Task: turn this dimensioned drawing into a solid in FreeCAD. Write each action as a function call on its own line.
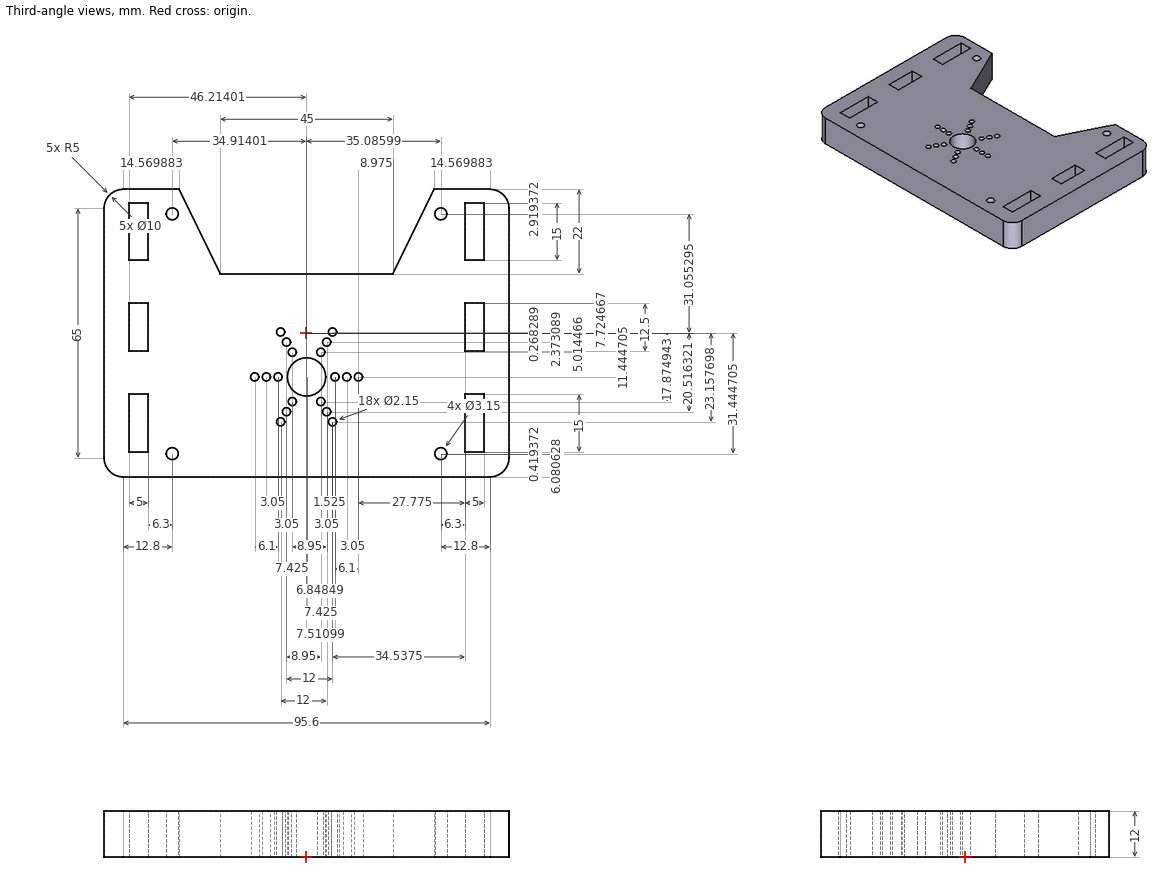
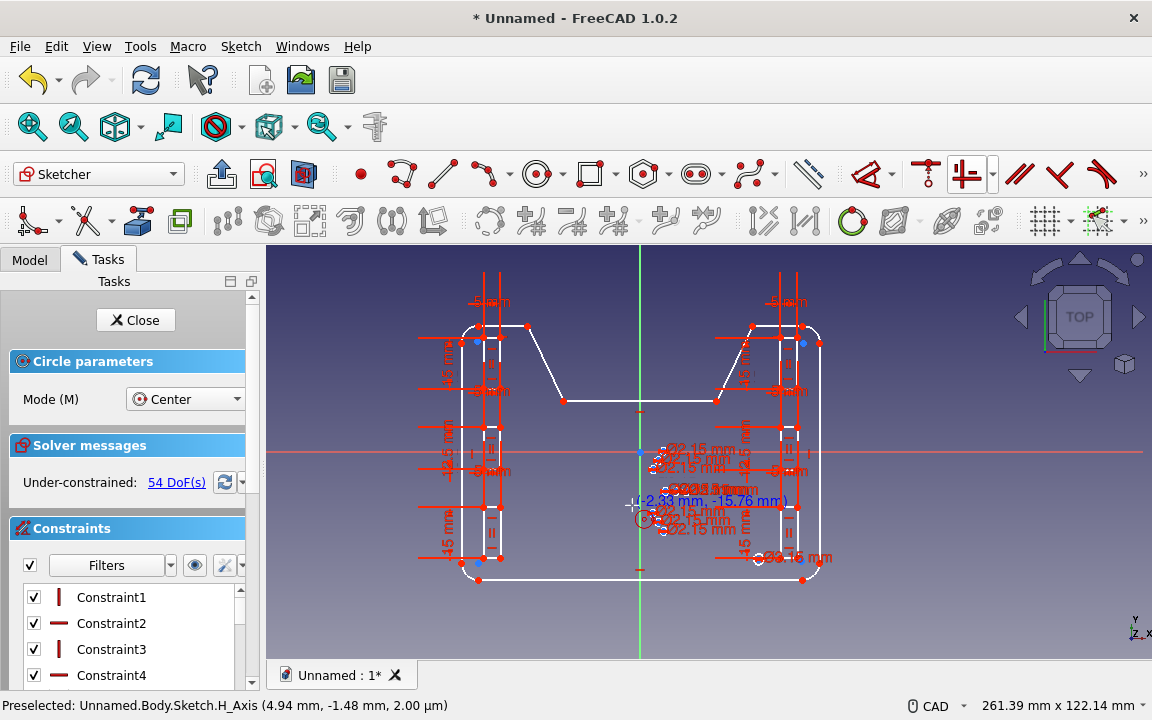
click(623, 522)
move(625, 519)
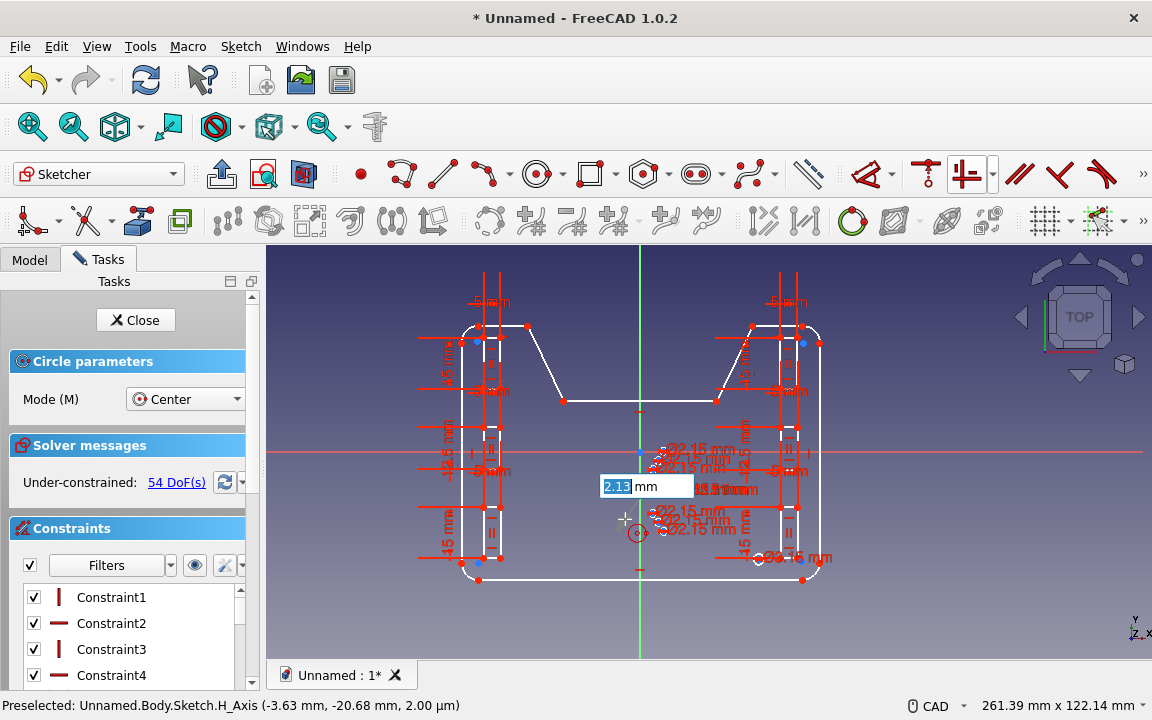
text(2.15)
key(Return)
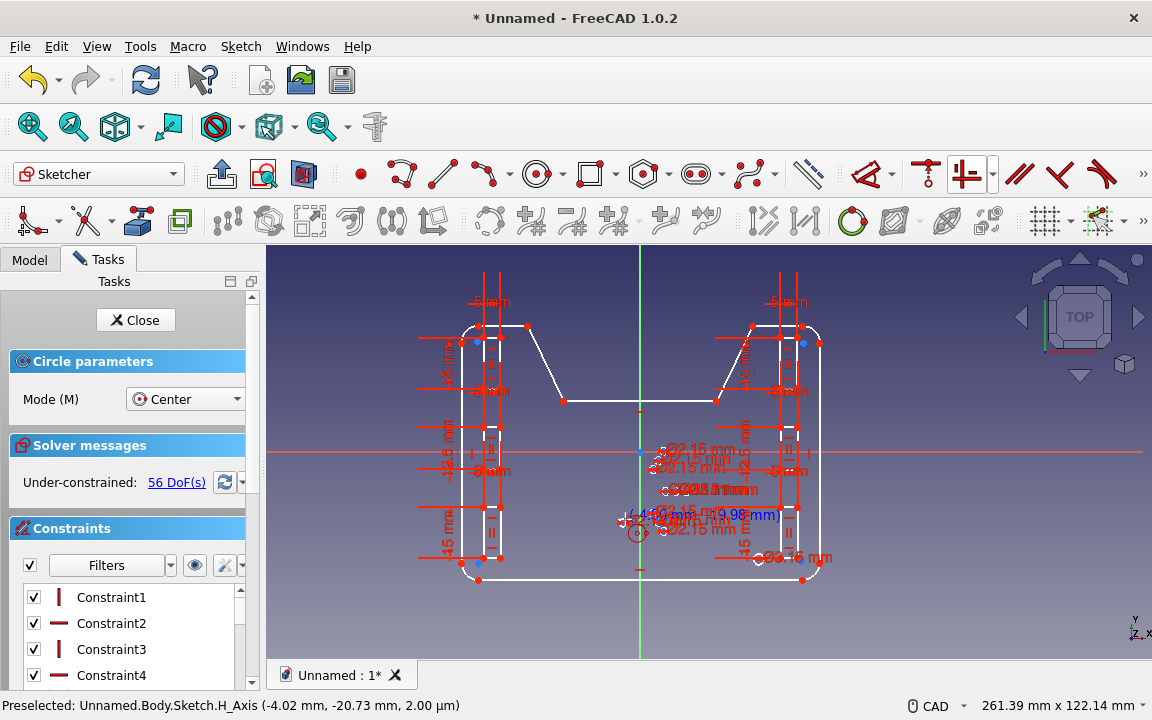
scroll(618, 531, up, 10)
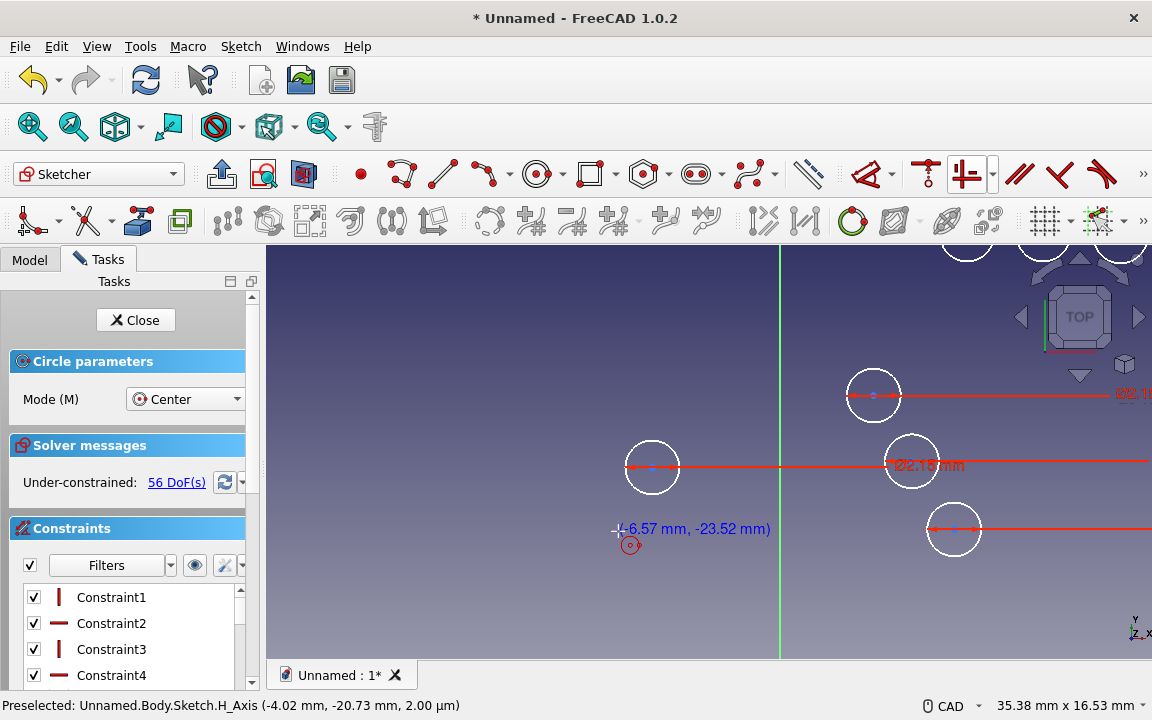
scroll(618, 531, down, 10)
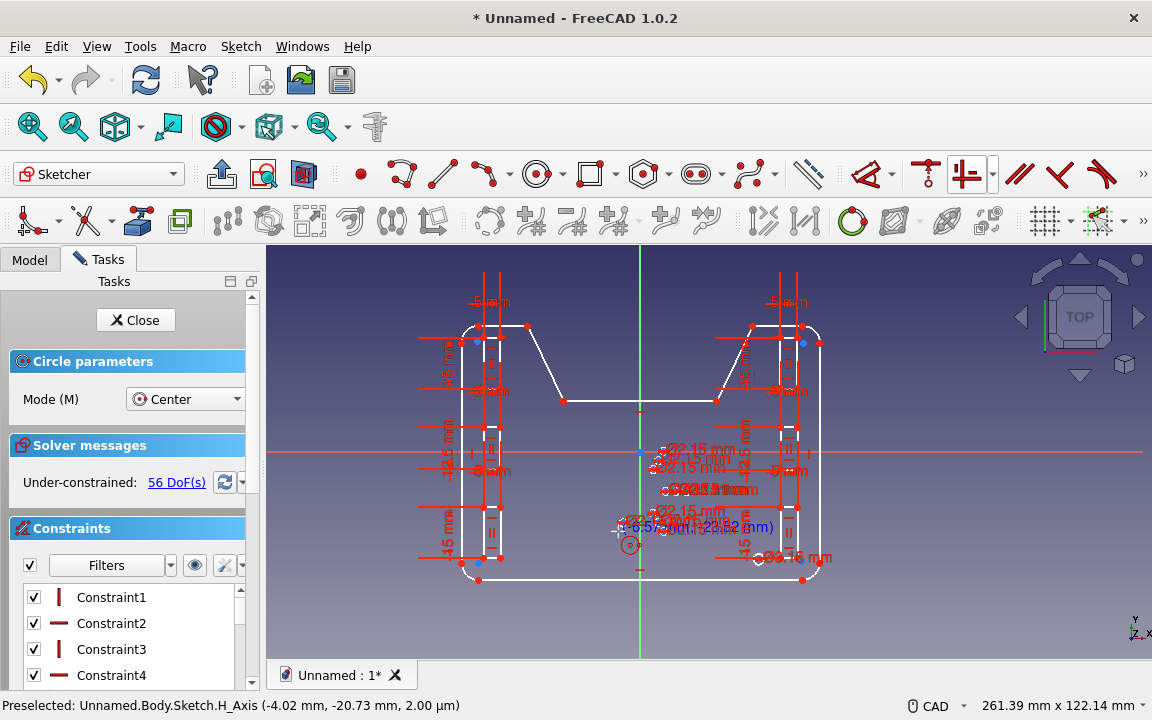
scroll(618, 531, up, 5)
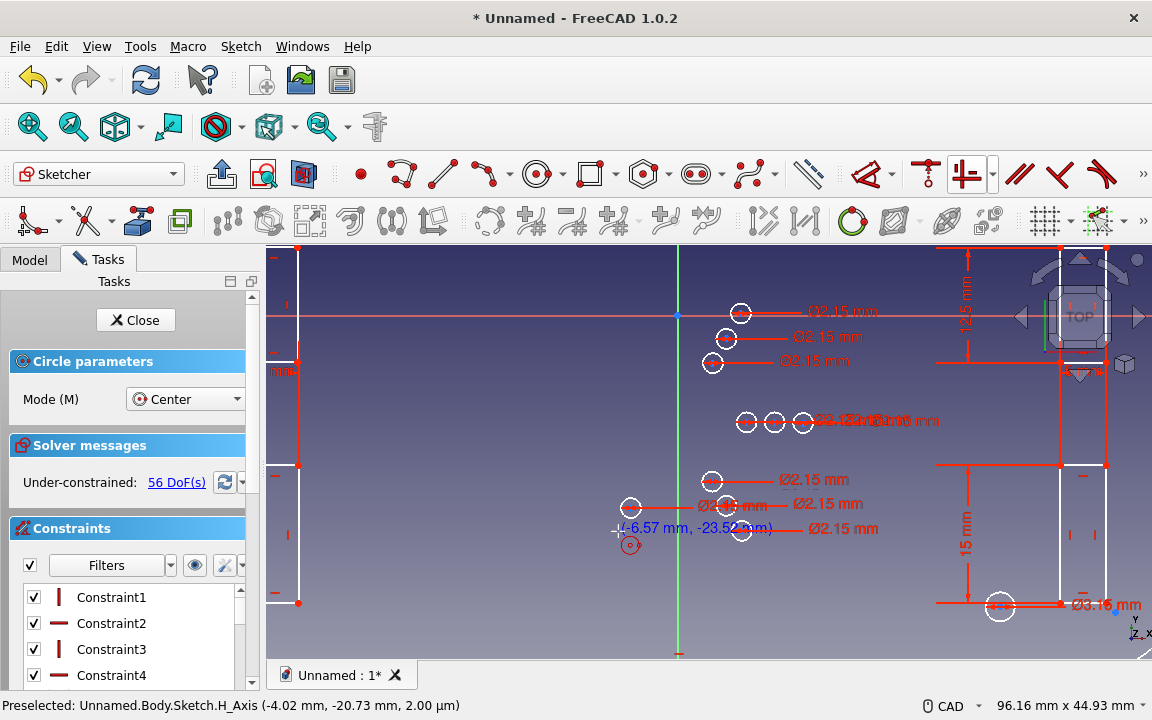
click(616, 529)
move(609, 522)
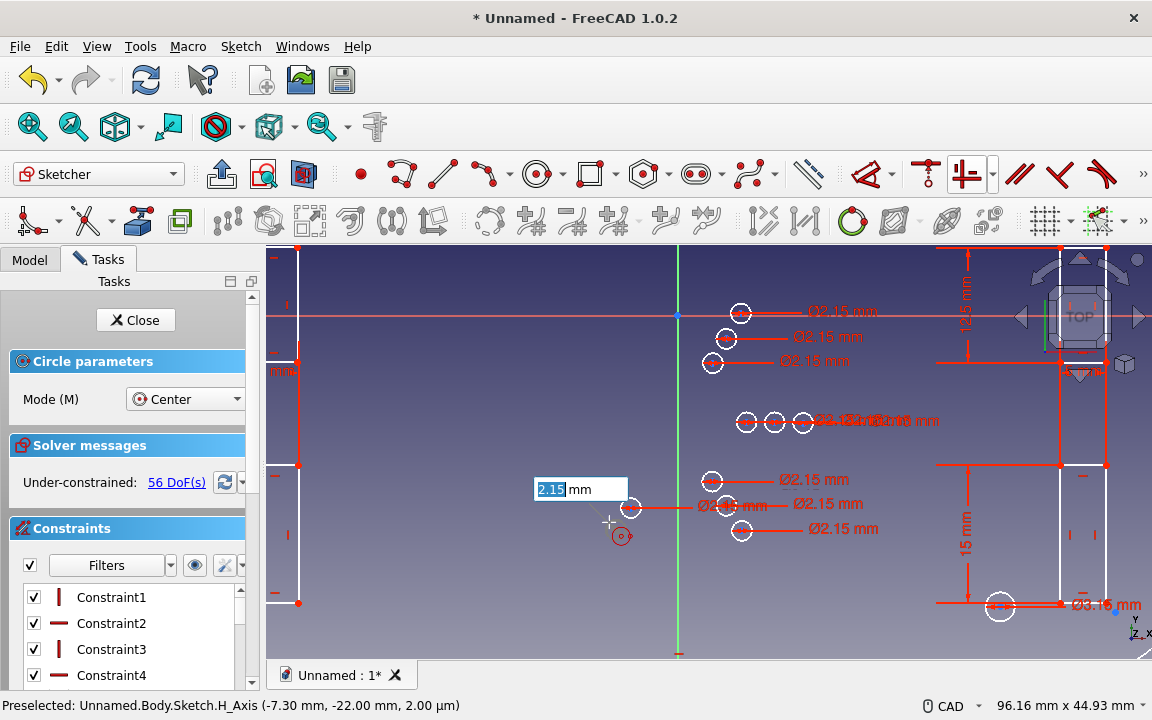
text(2.15)
key(Return)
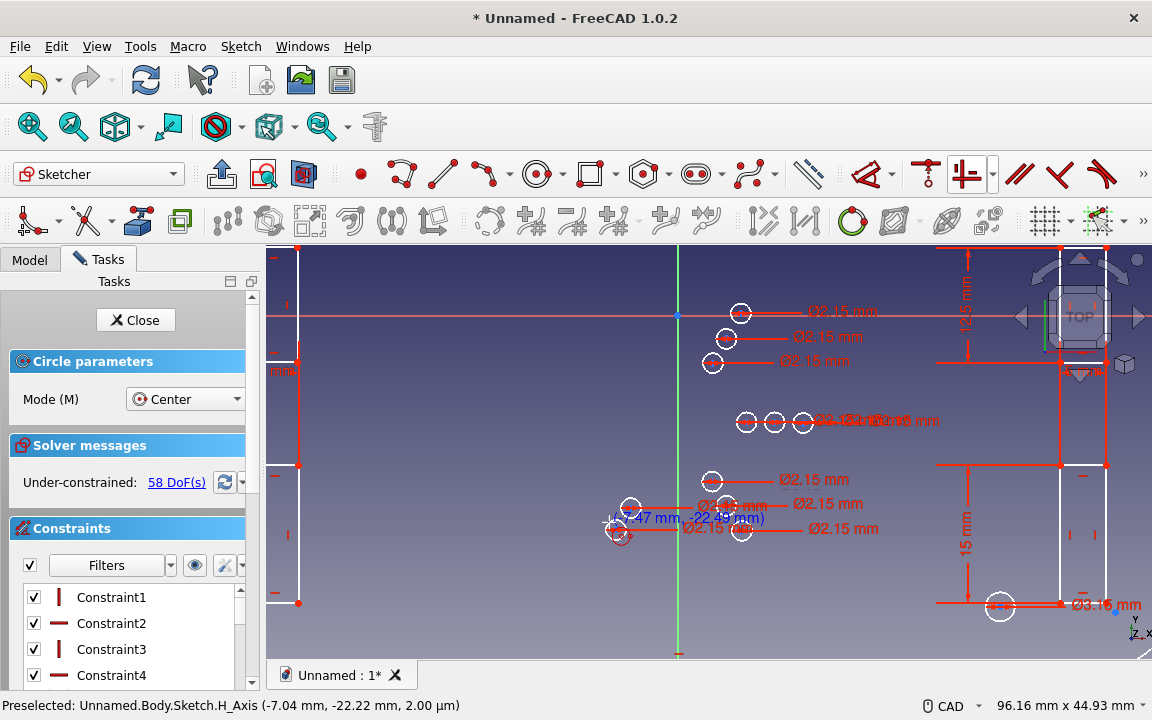
scroll(644, 481, up, 5)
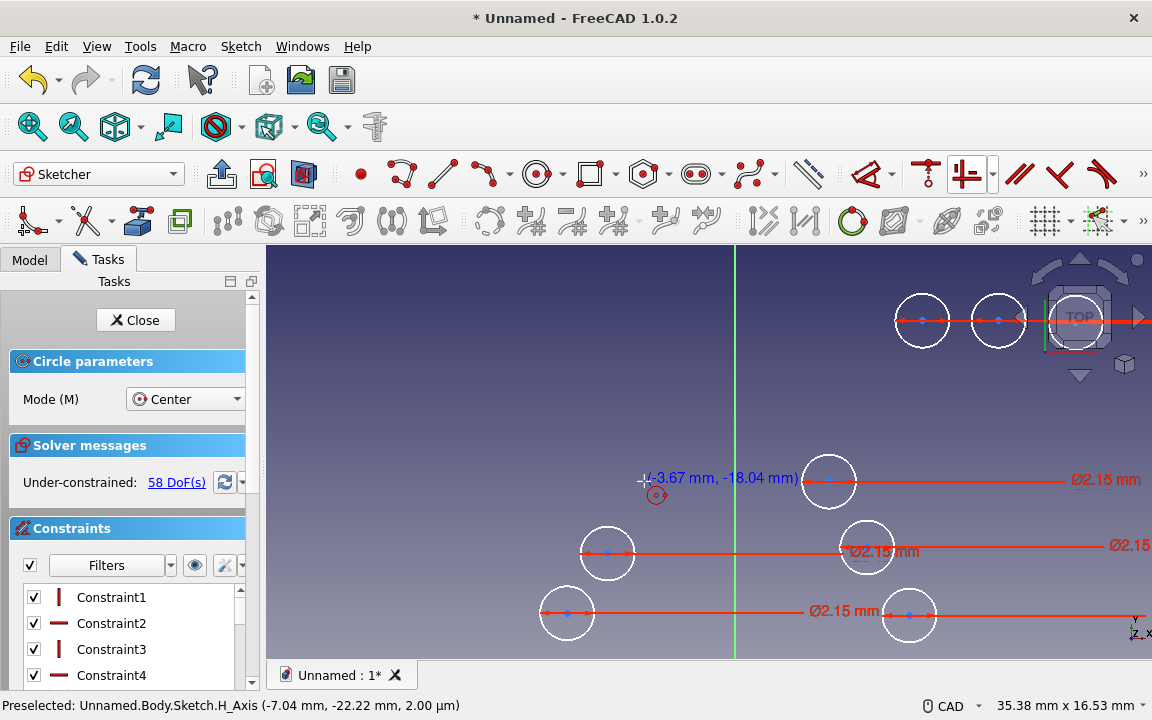
scroll(625, 518, down, 10)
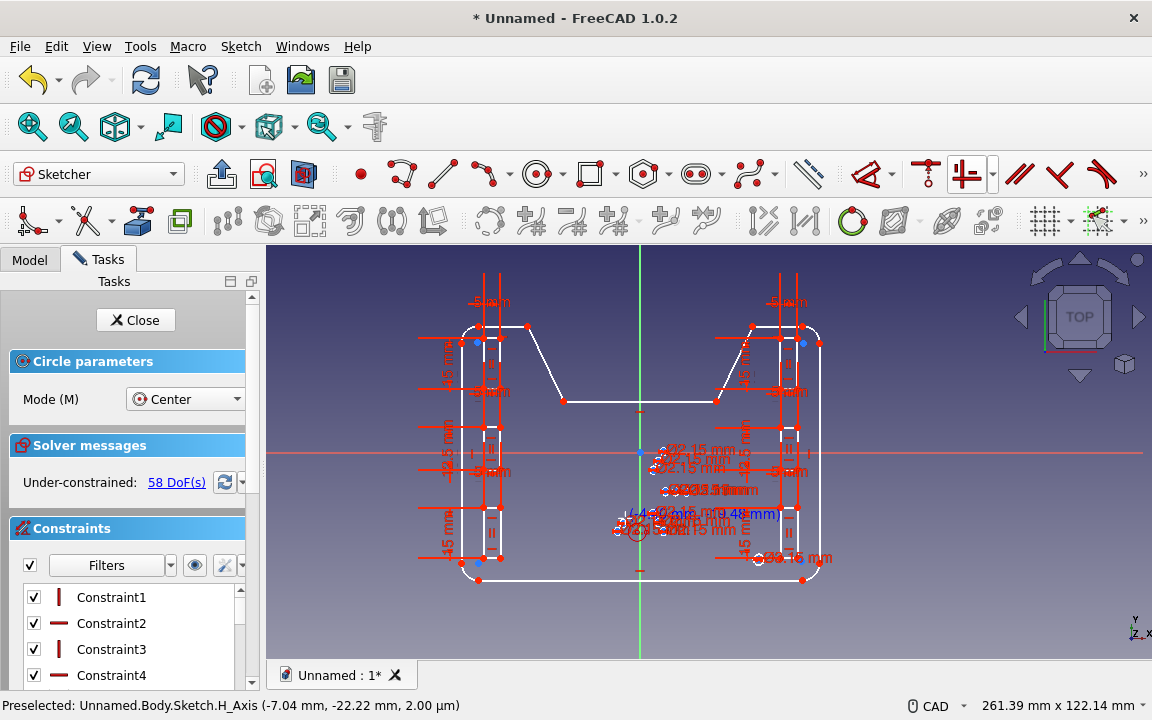
scroll(628, 513, up, 5)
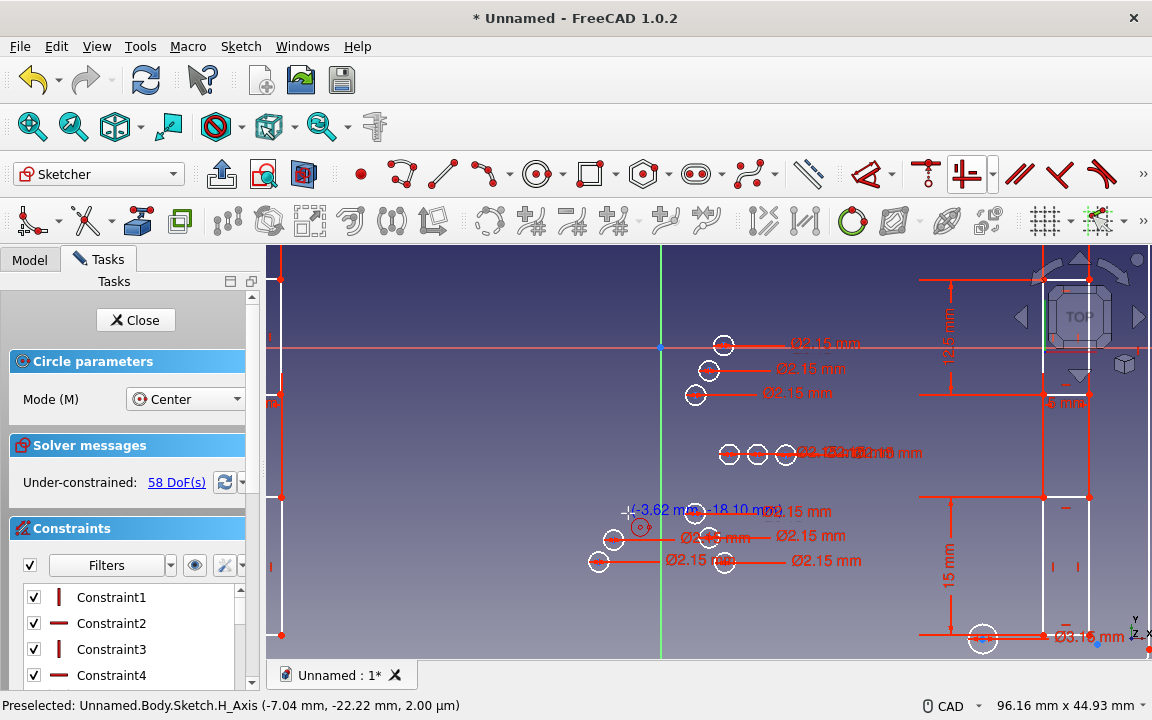
click(627, 513)
move(634, 506)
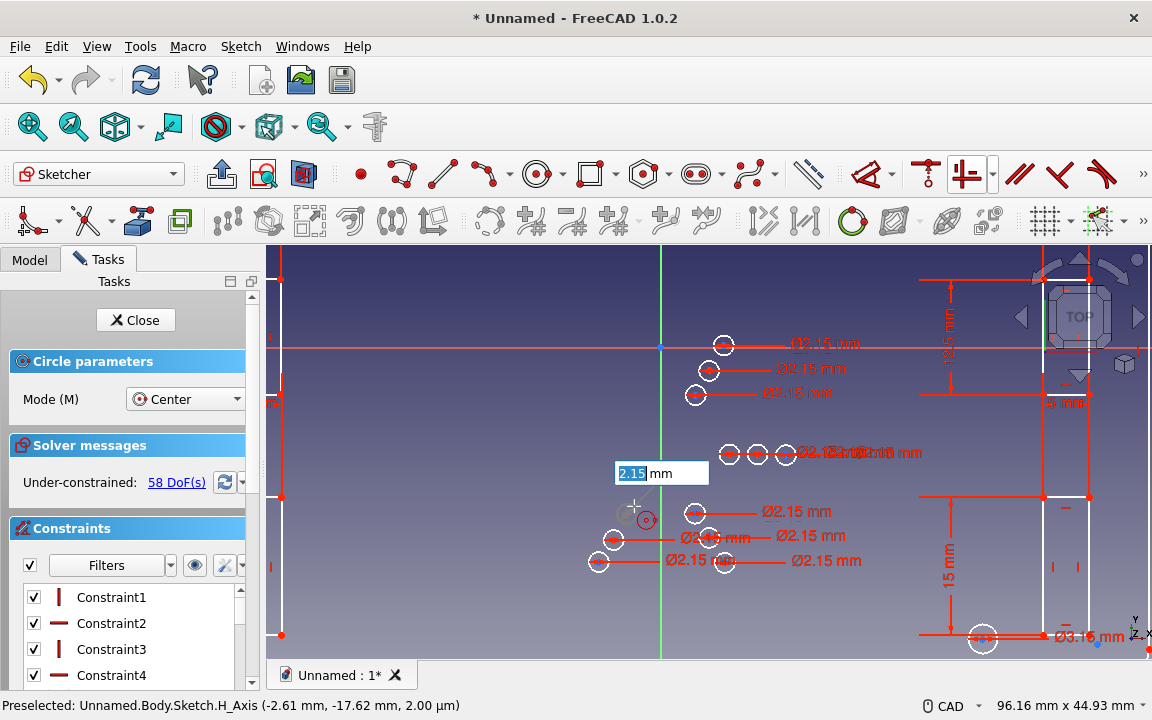
text(2.15)
key(Return)